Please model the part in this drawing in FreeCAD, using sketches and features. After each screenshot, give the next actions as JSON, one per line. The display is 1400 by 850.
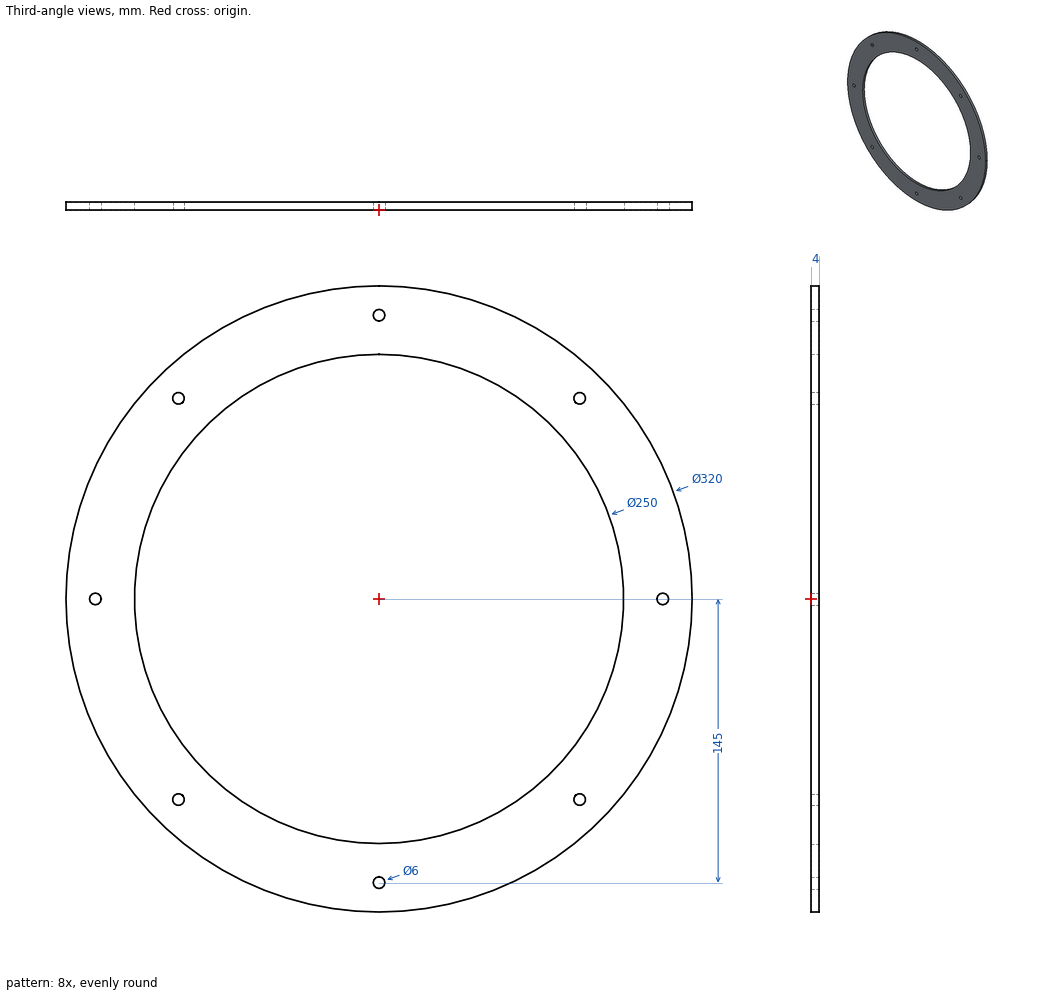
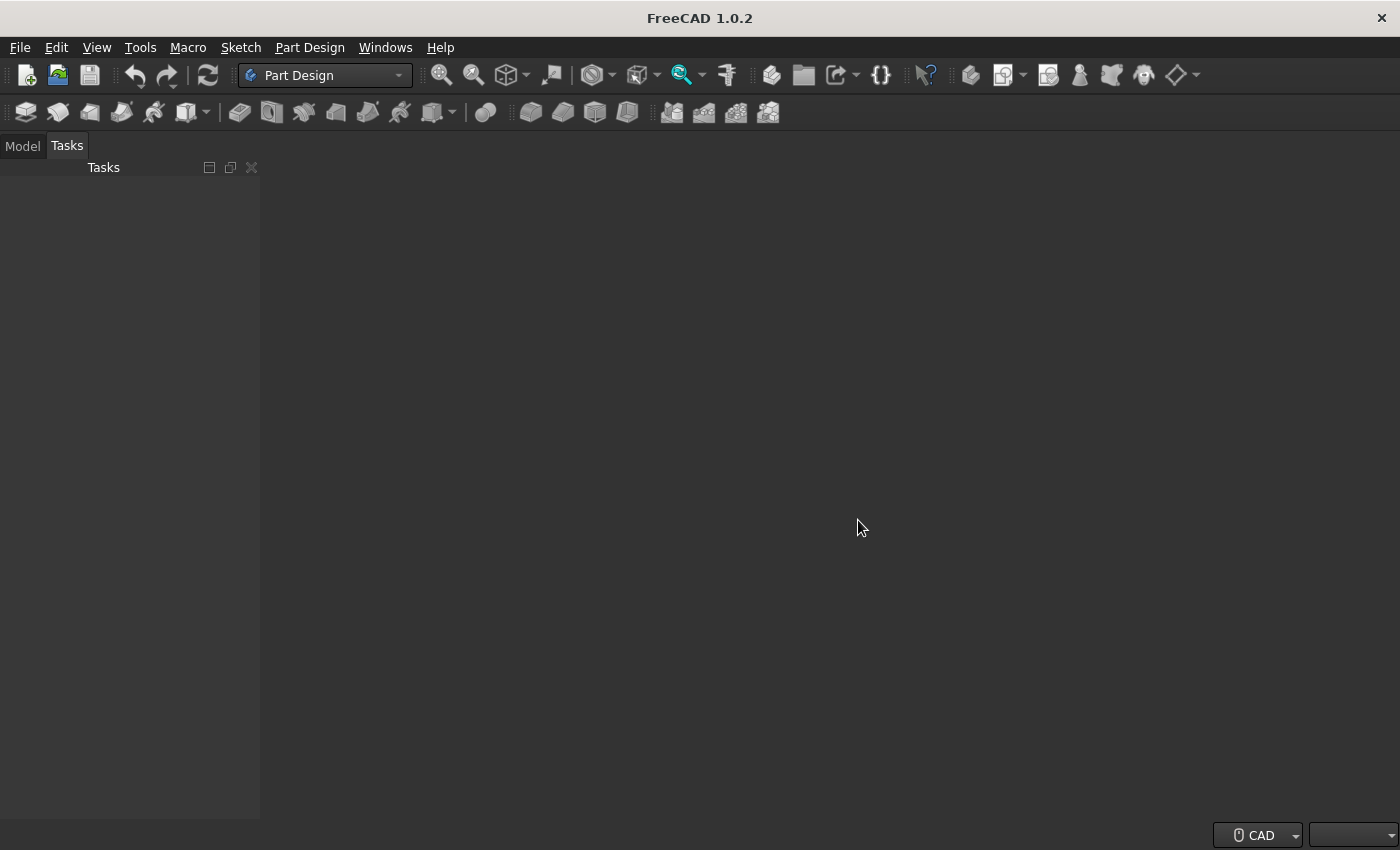
{"action": "left_click", "coordinate": [26, 76]}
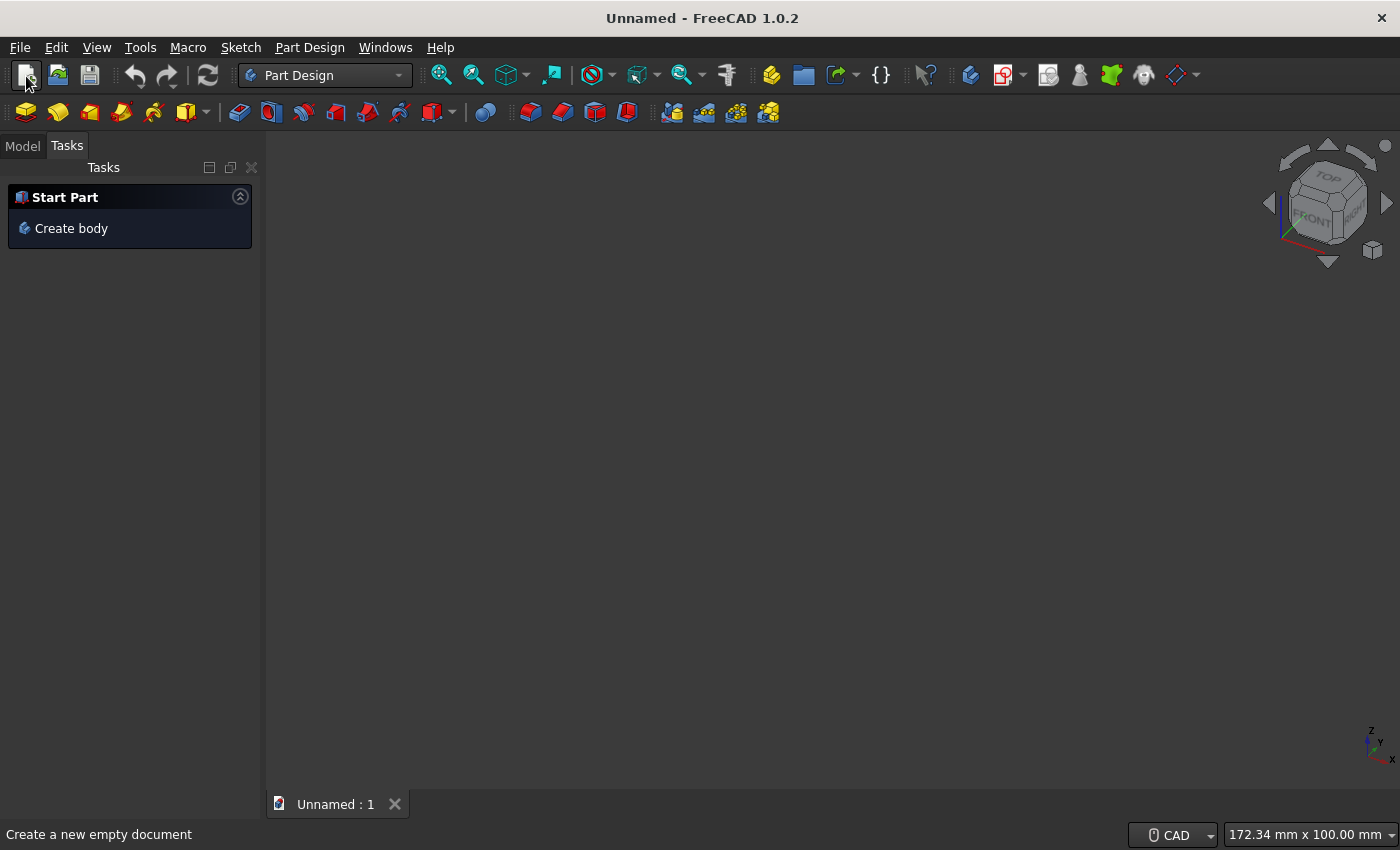
{"action": "left_click", "coordinate": [1004, 76]}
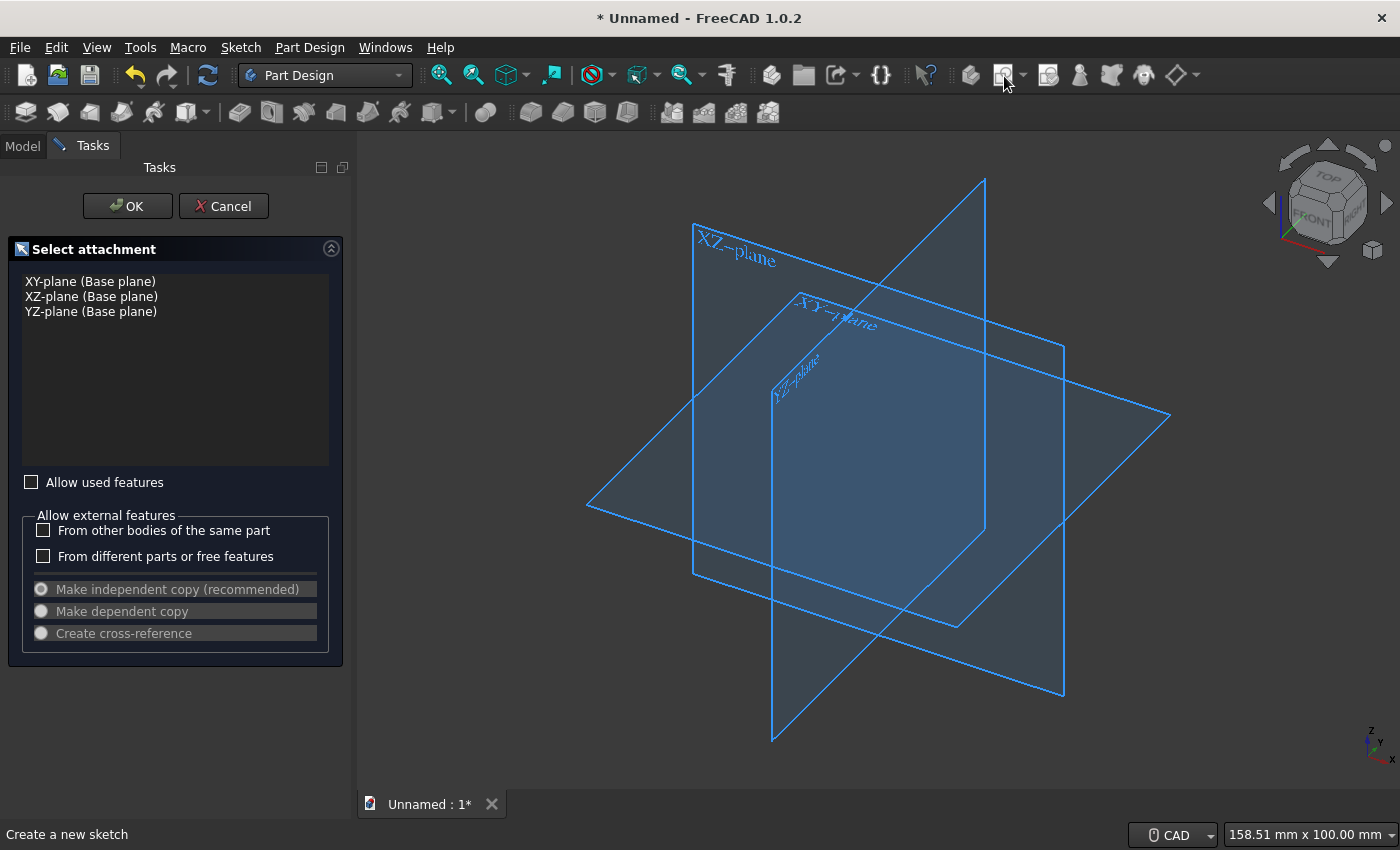
{"action": "left_click", "coordinate": [82, 296]}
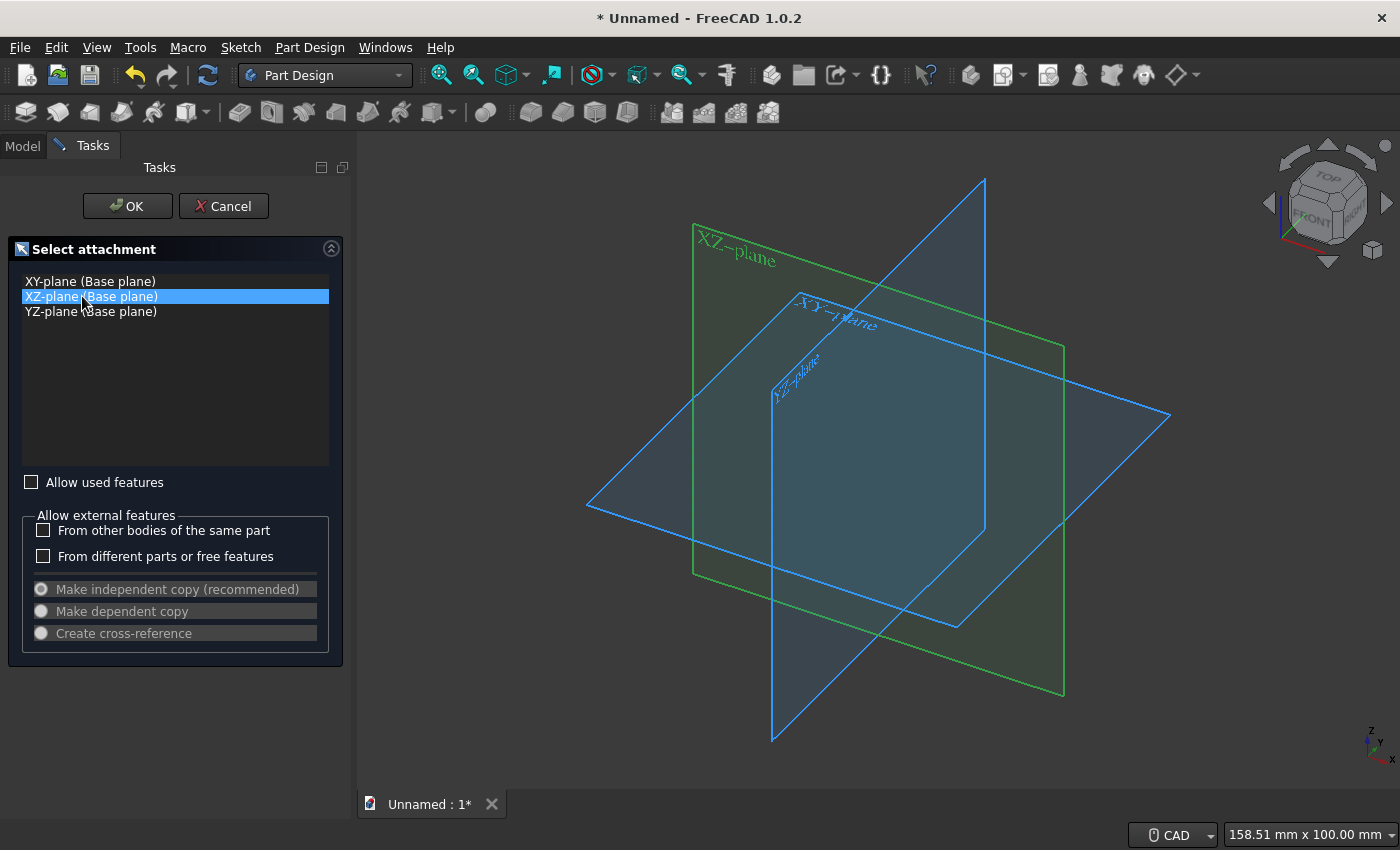
{"action": "left_click", "coordinate": [128, 206]}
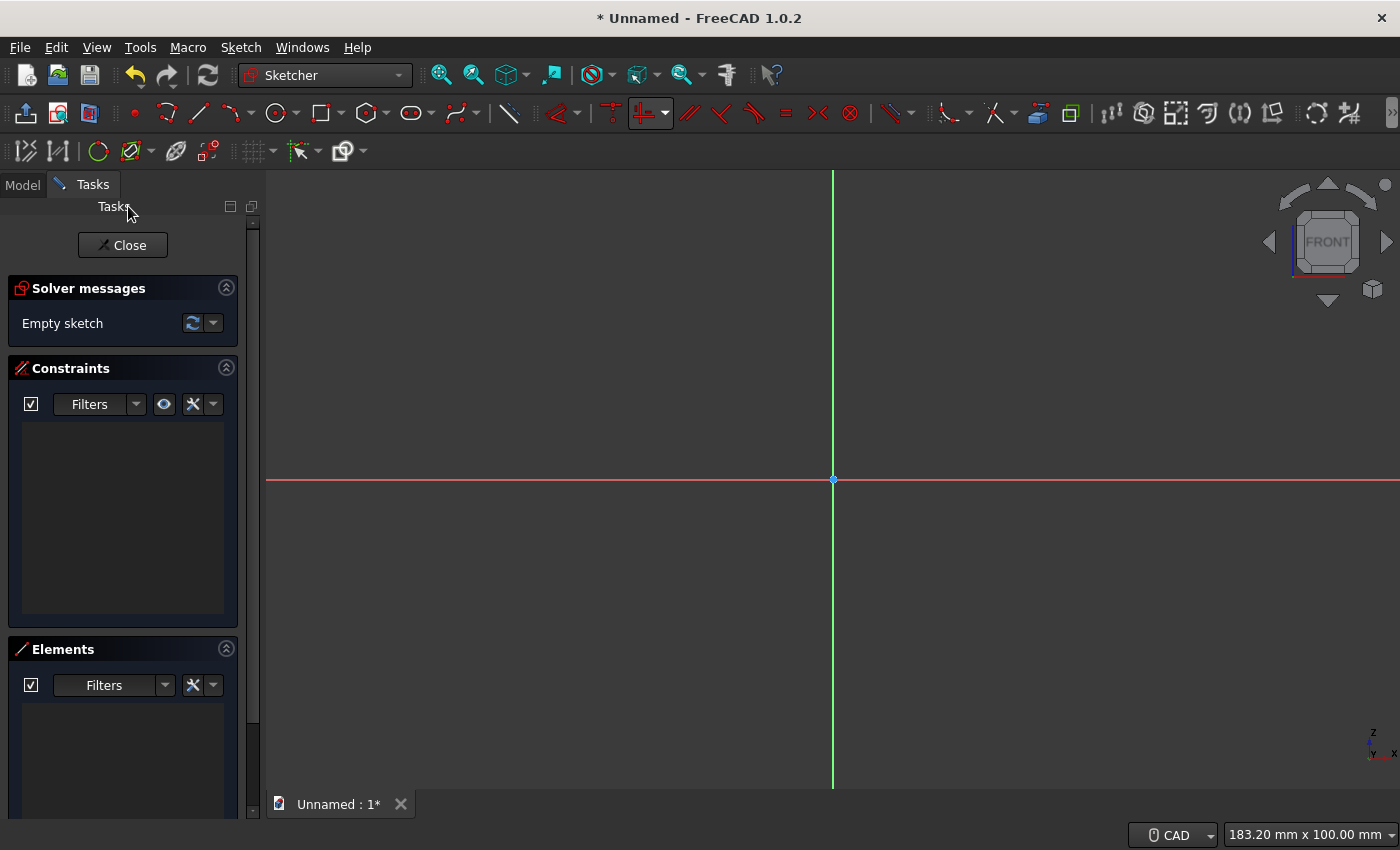
{"action": "scroll", "coordinate": [747, 480], "scroll_direction": "down", "scroll_amount": 8}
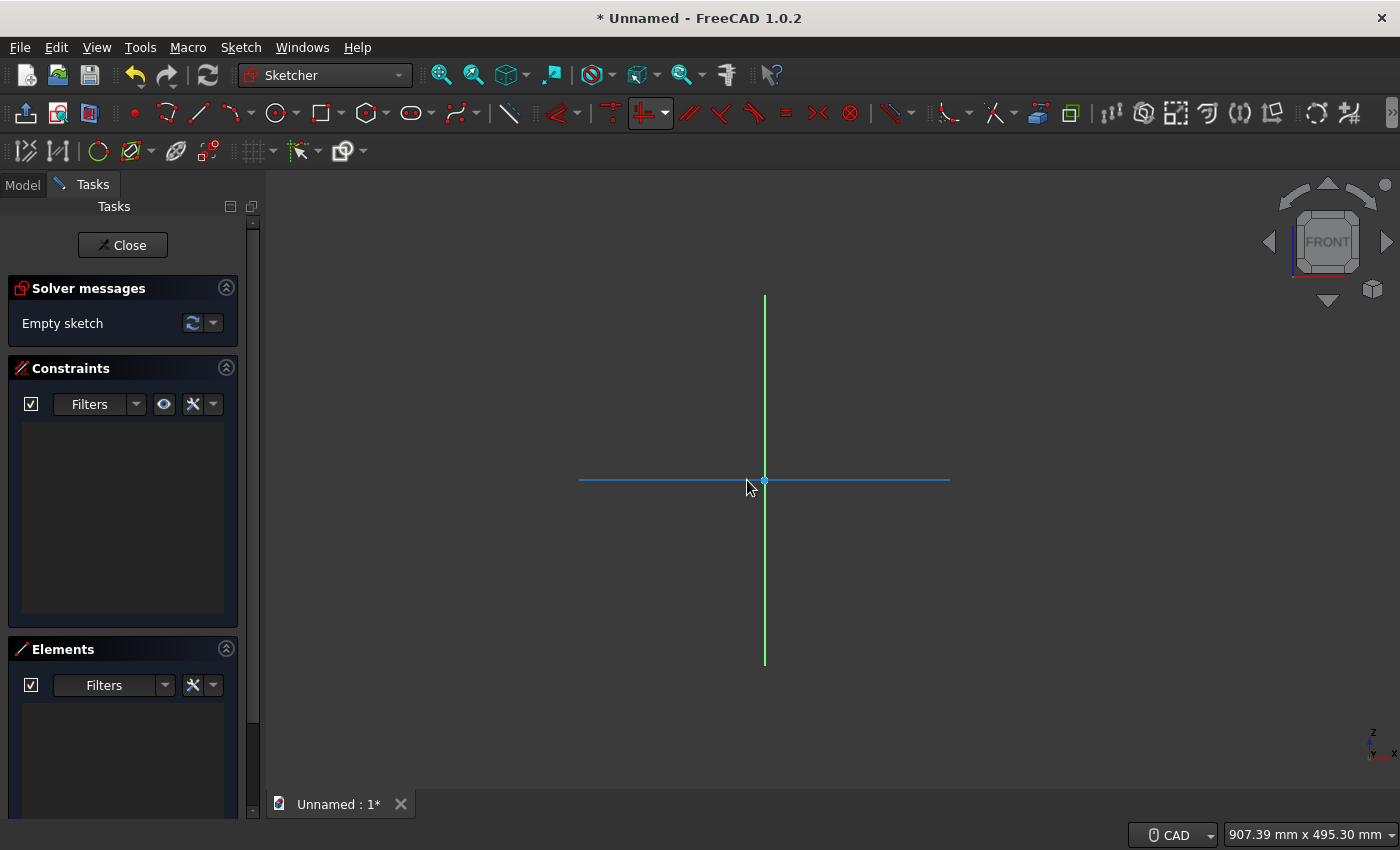
{"action": "key", "text": "g c"}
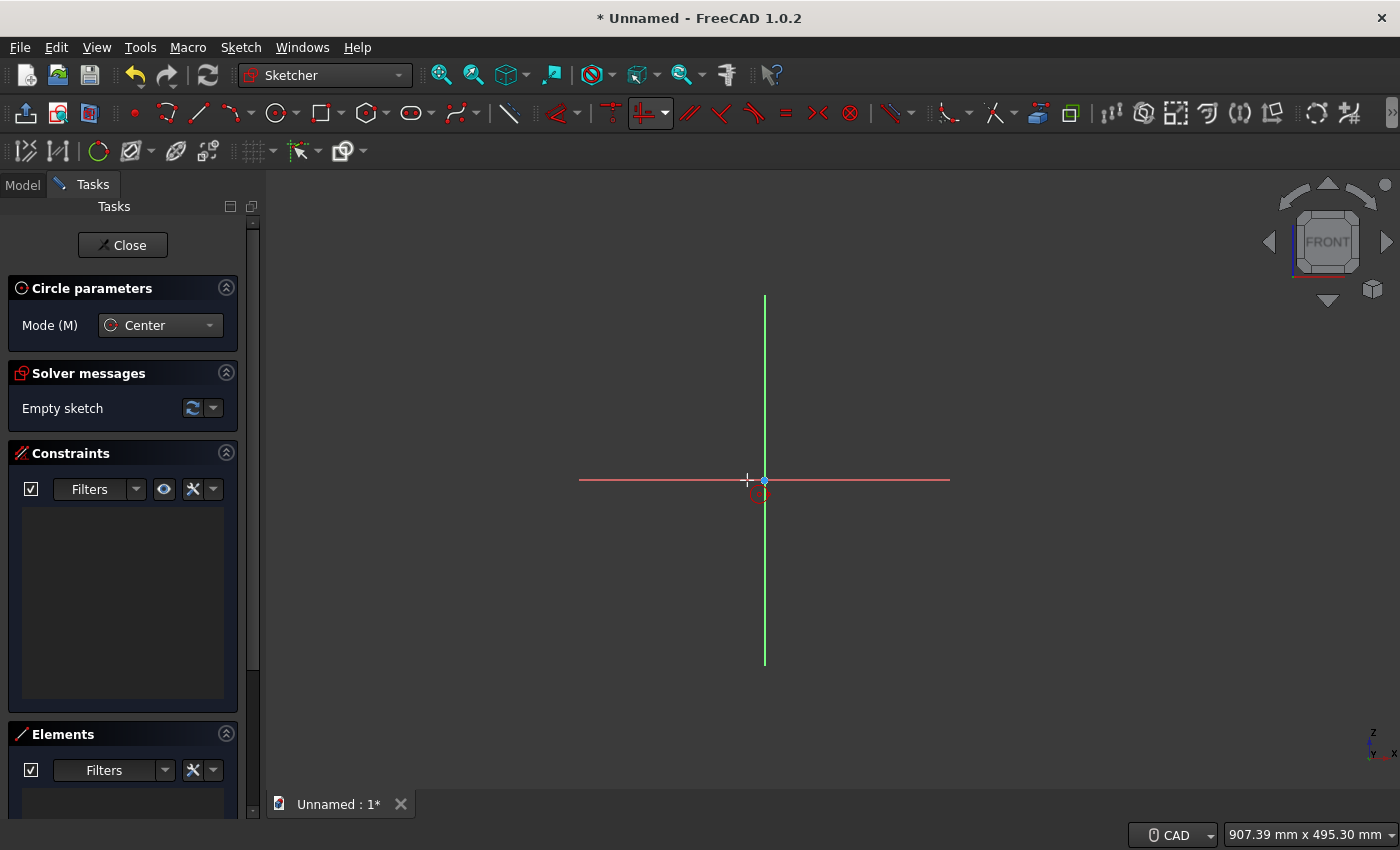
{"action": "left_click", "coordinate": [765, 480]}
{"action": "mouse_move", "coordinate": [906, 339]}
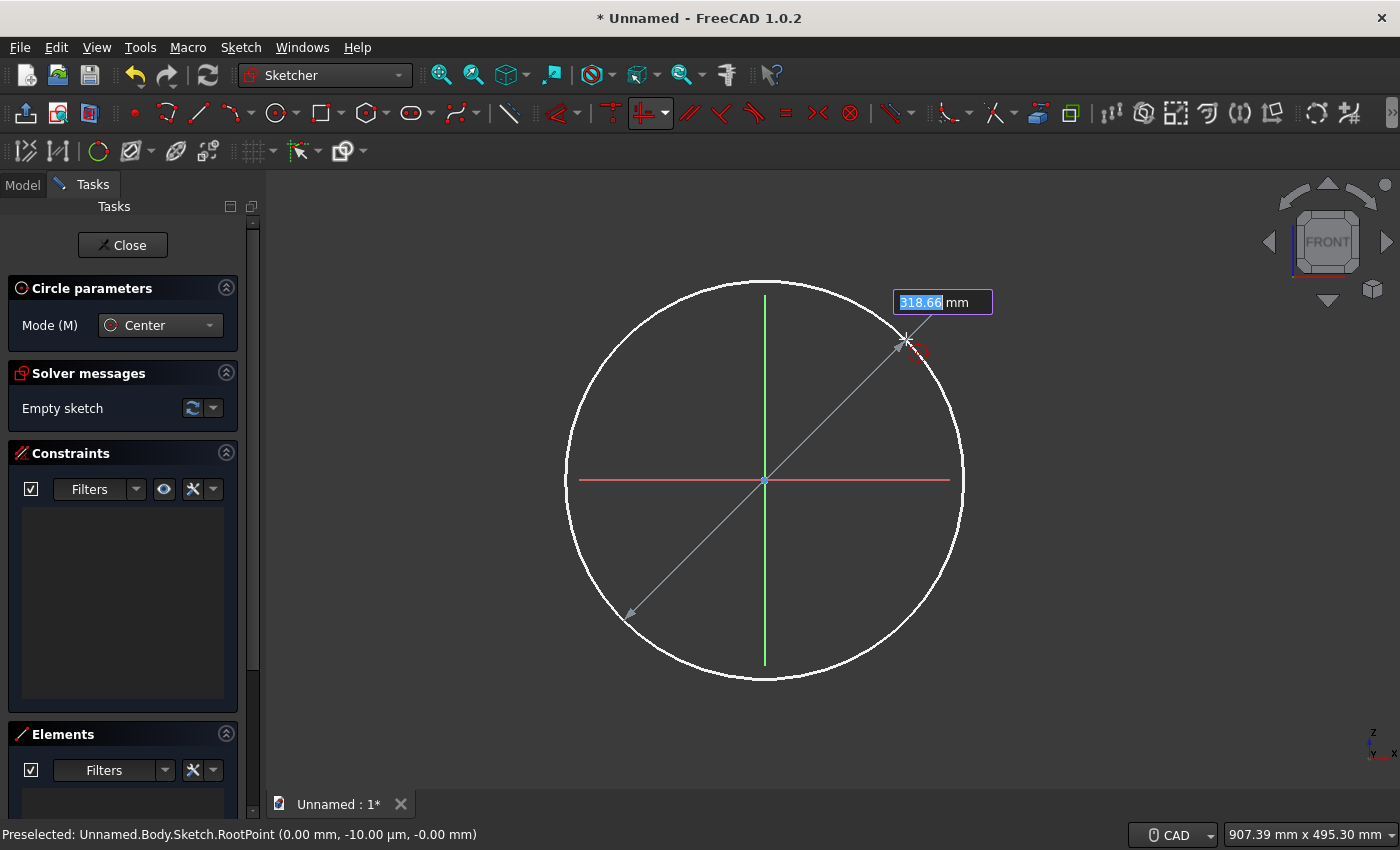
{"action": "type", "text": "320"}
{"action": "key", "text": "Return"}